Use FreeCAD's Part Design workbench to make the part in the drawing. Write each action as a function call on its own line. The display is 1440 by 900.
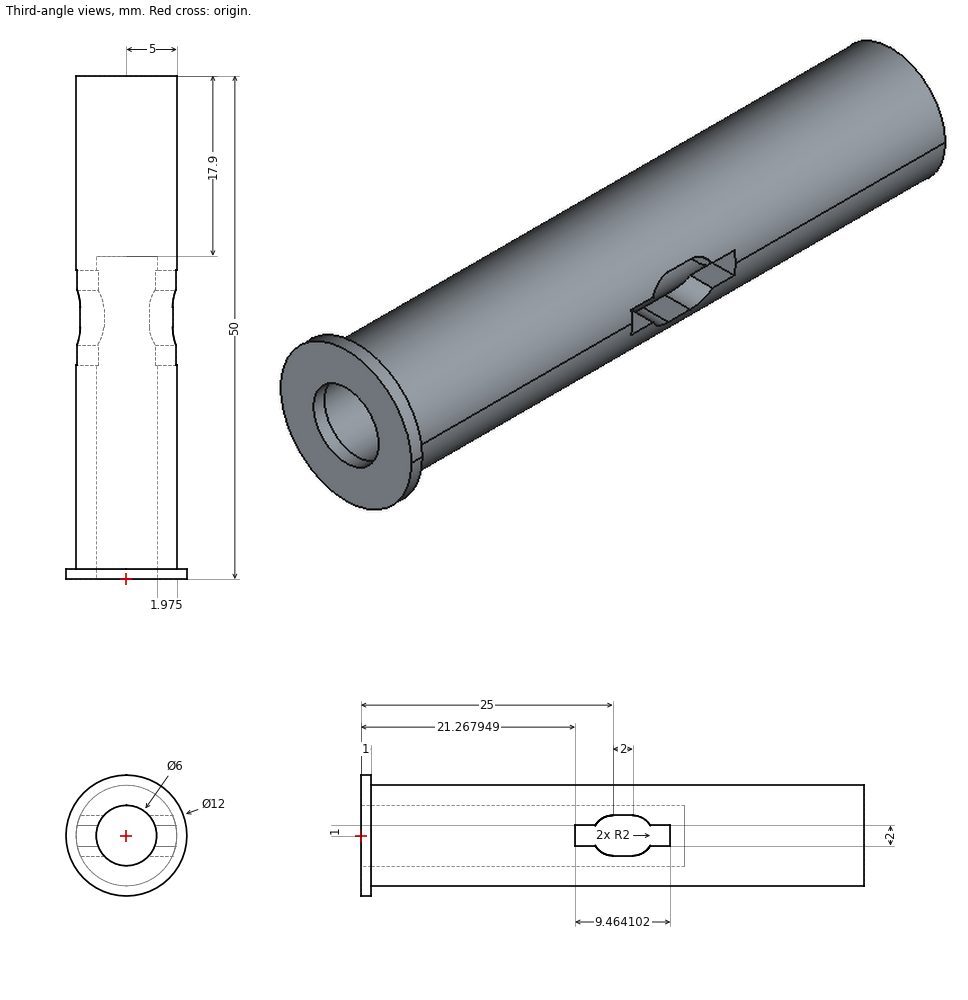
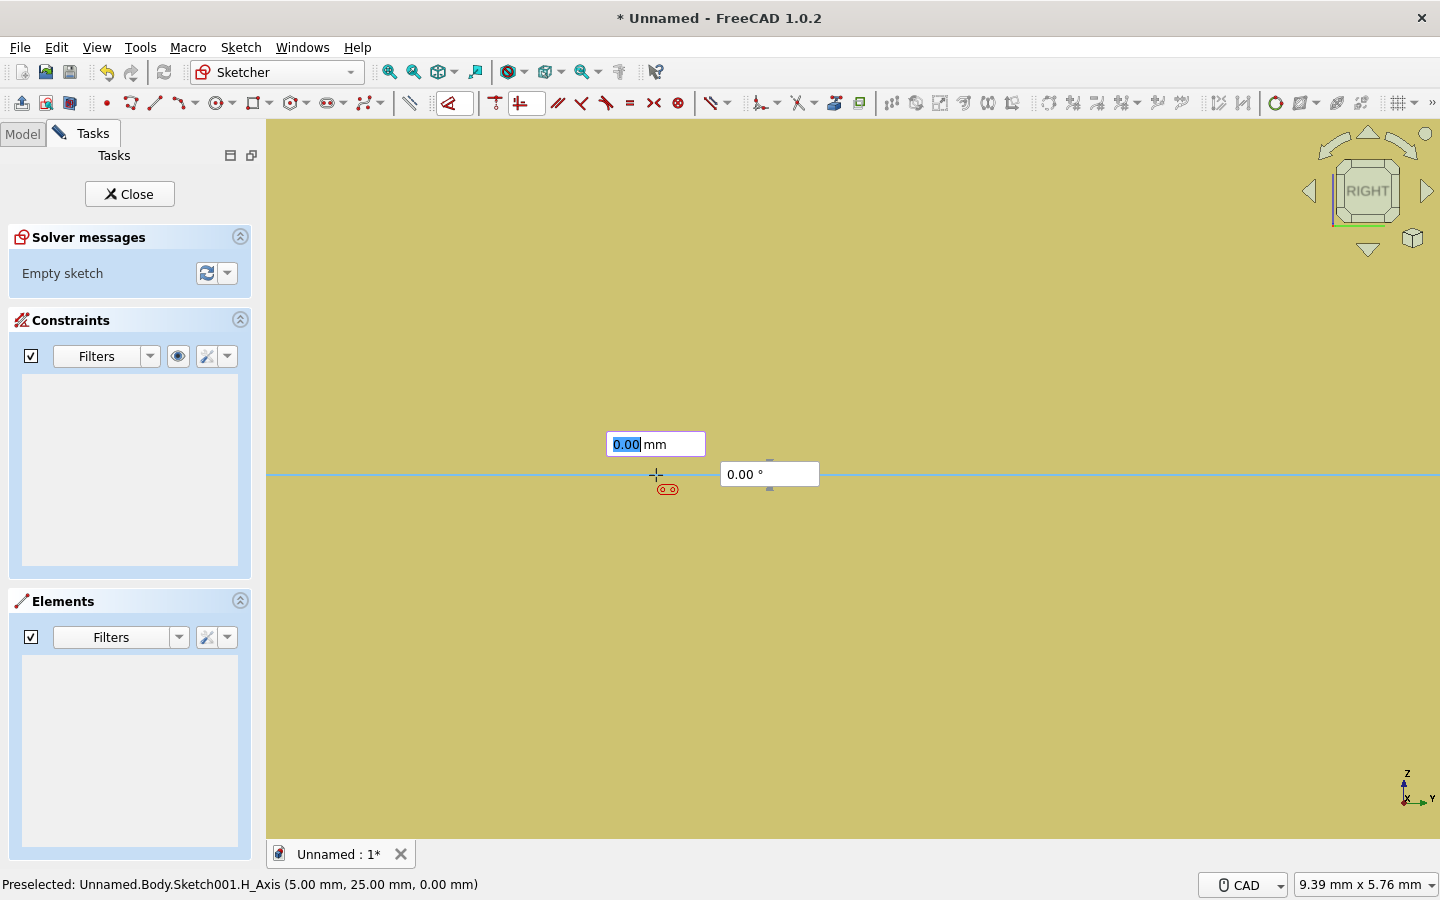
click(906, 466)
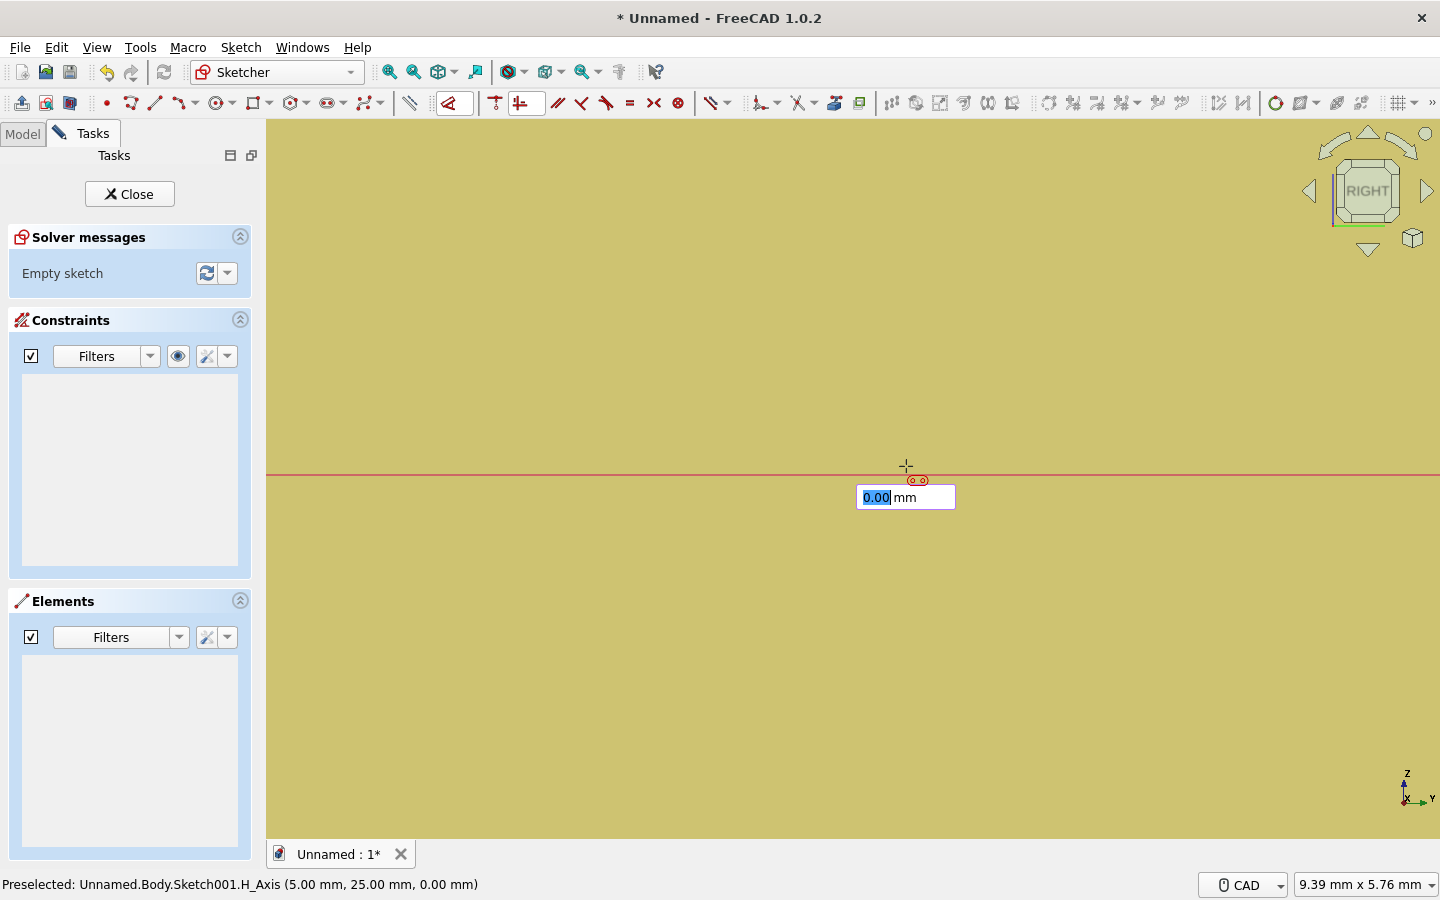
click(781, 725)
key(Escape)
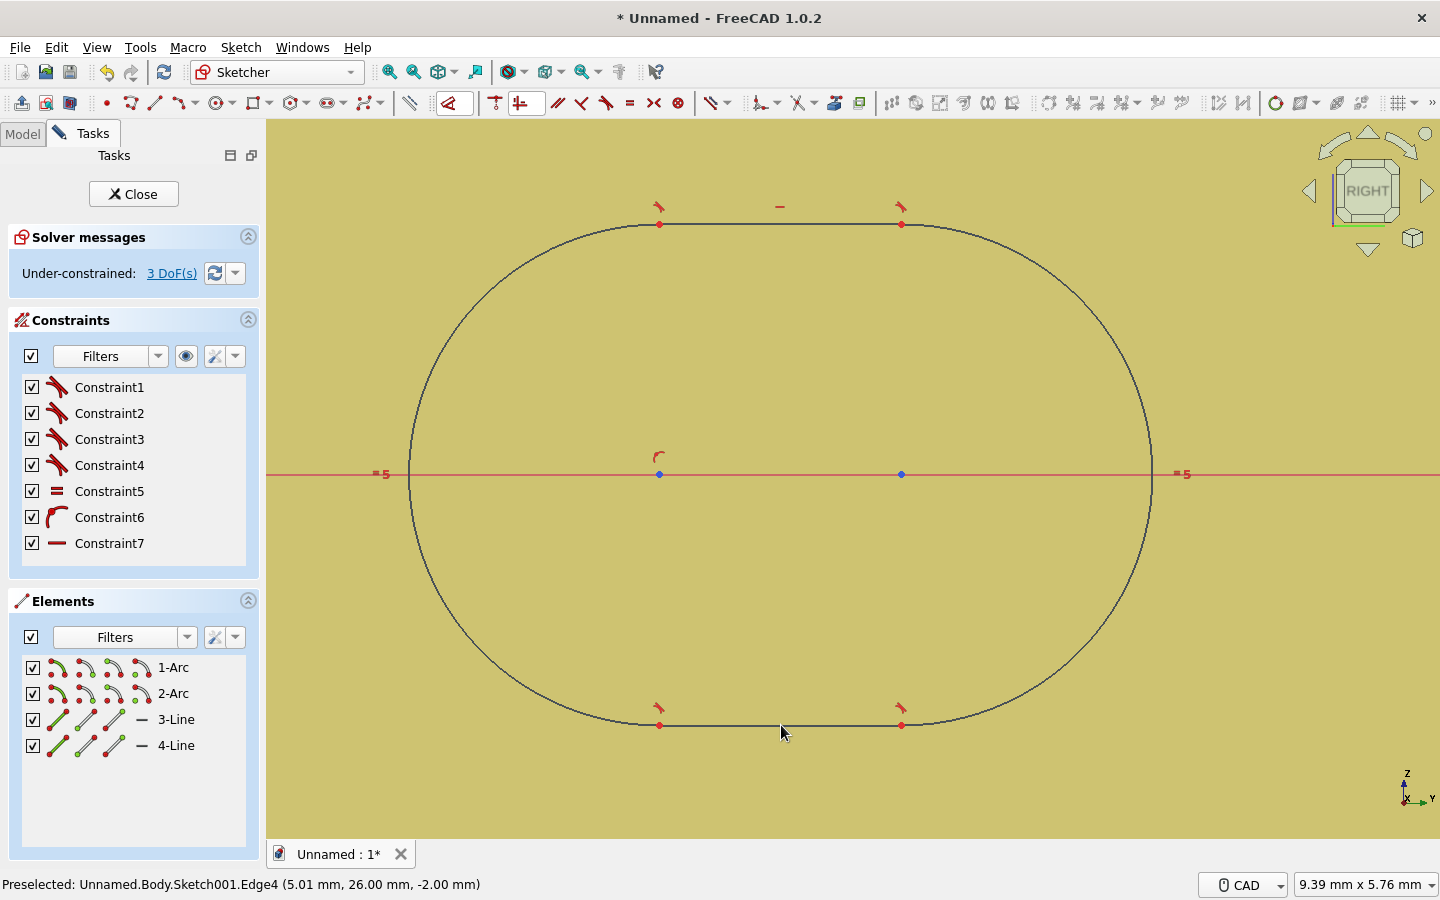
click(457, 328)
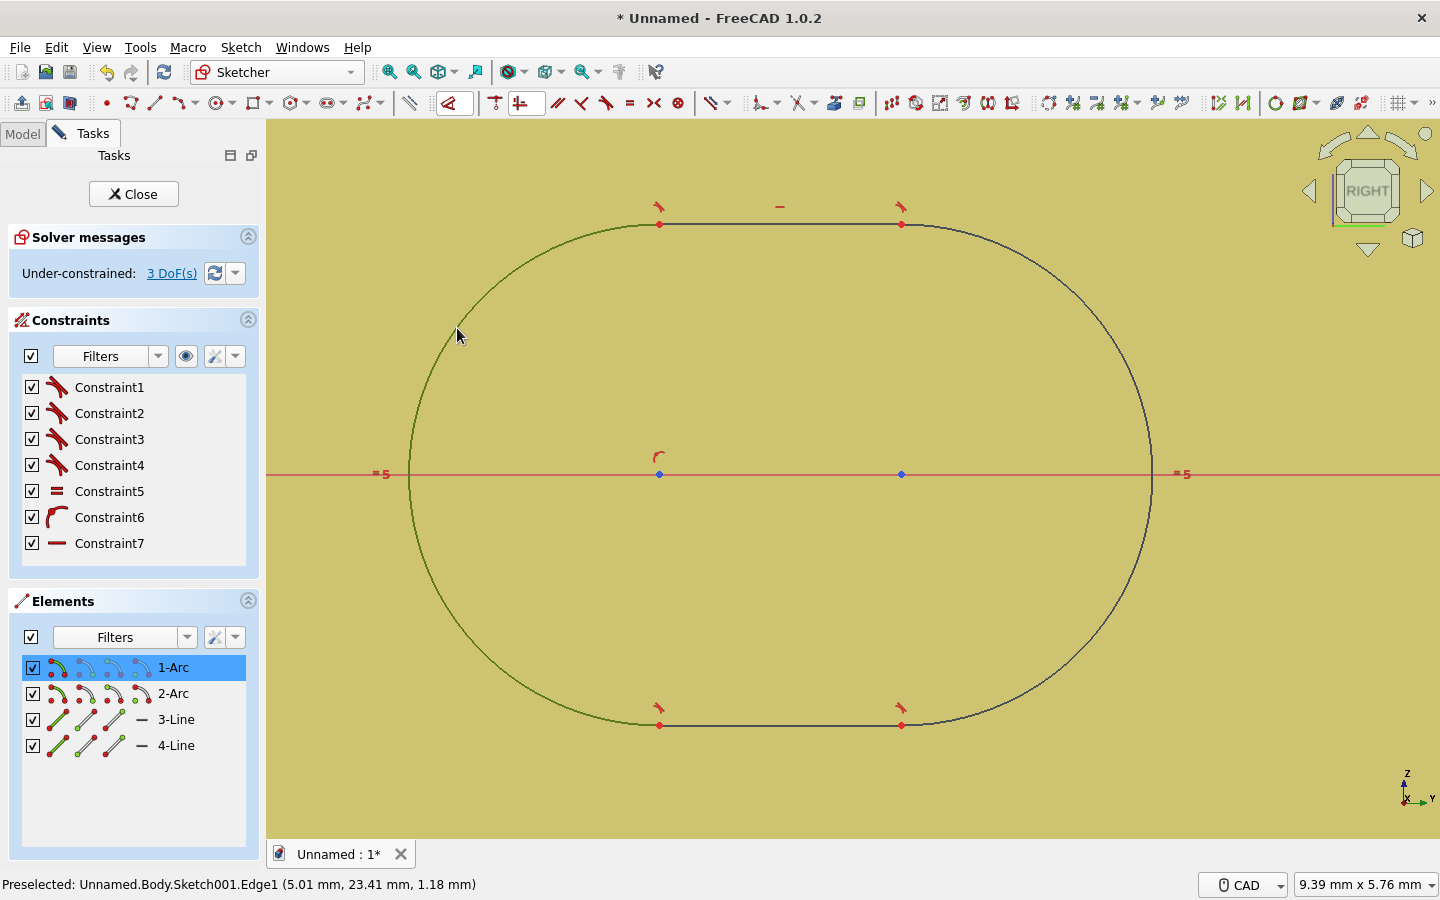
key(k)
key(r)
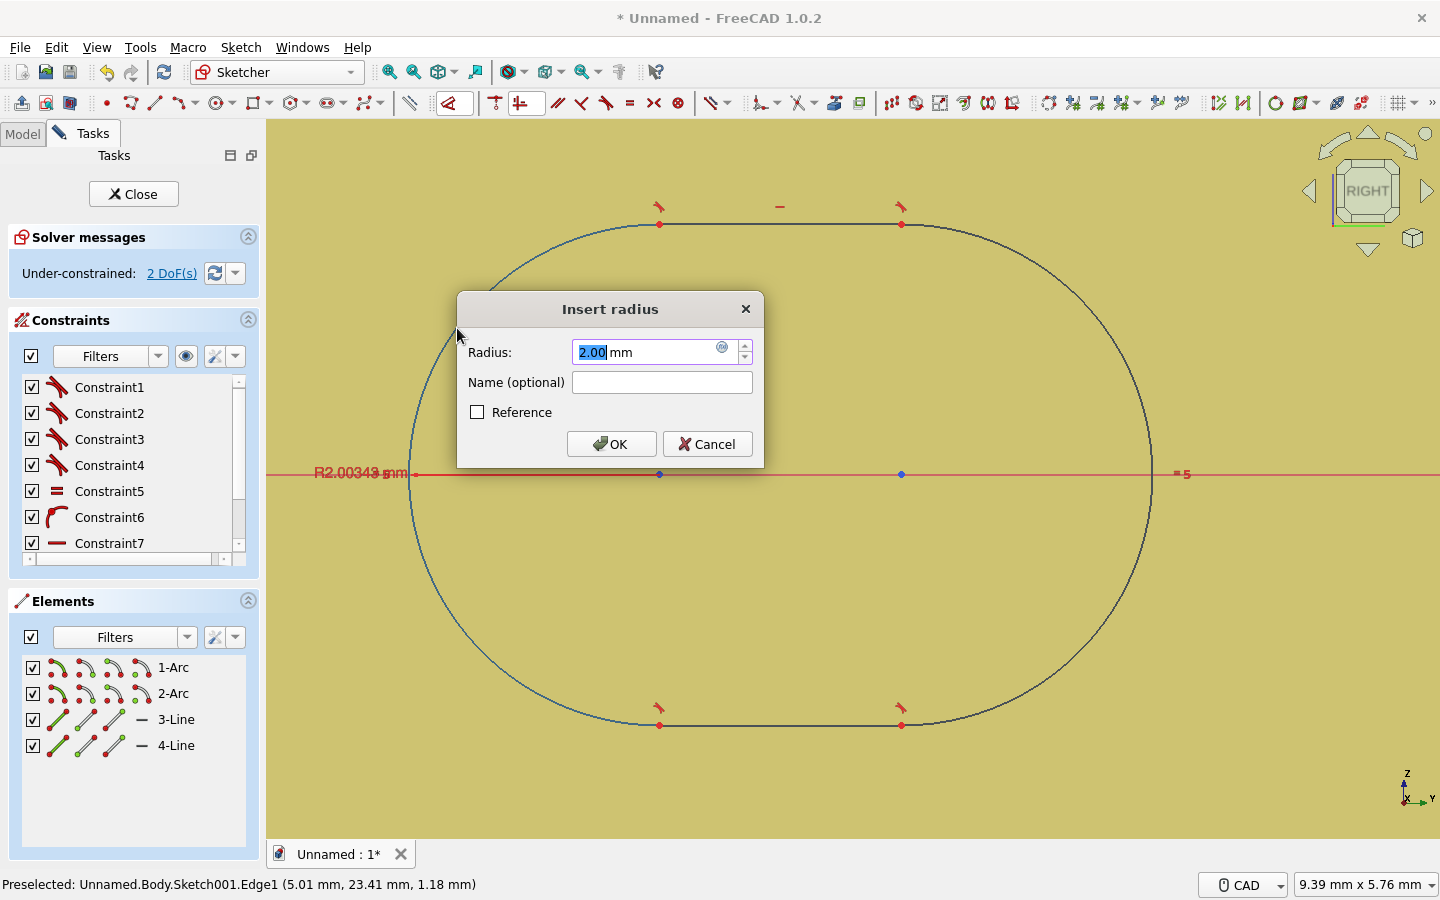
text(2)
key(Return)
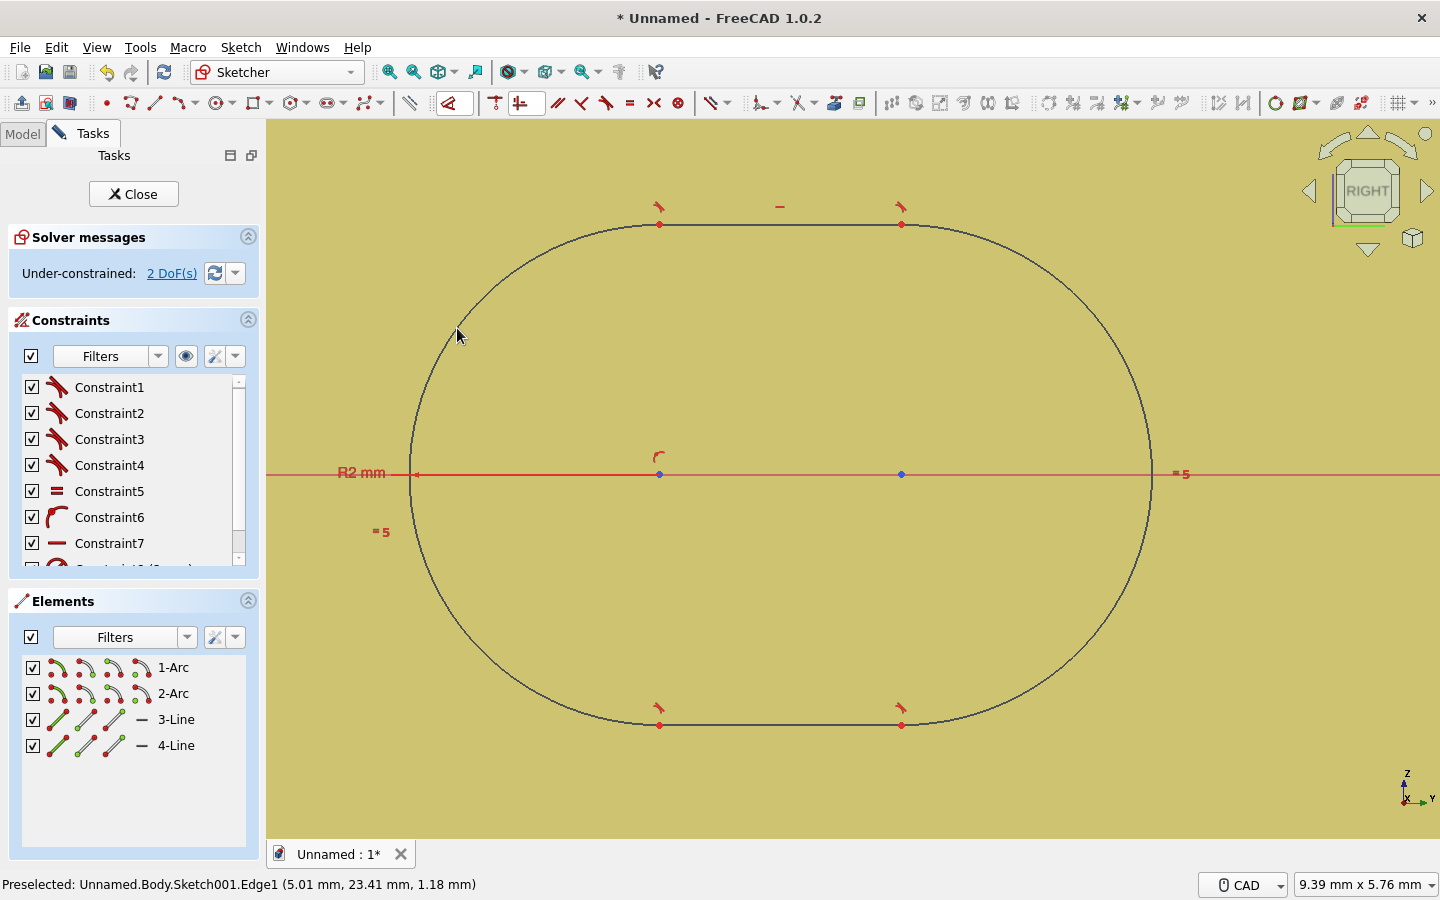
click(732, 225)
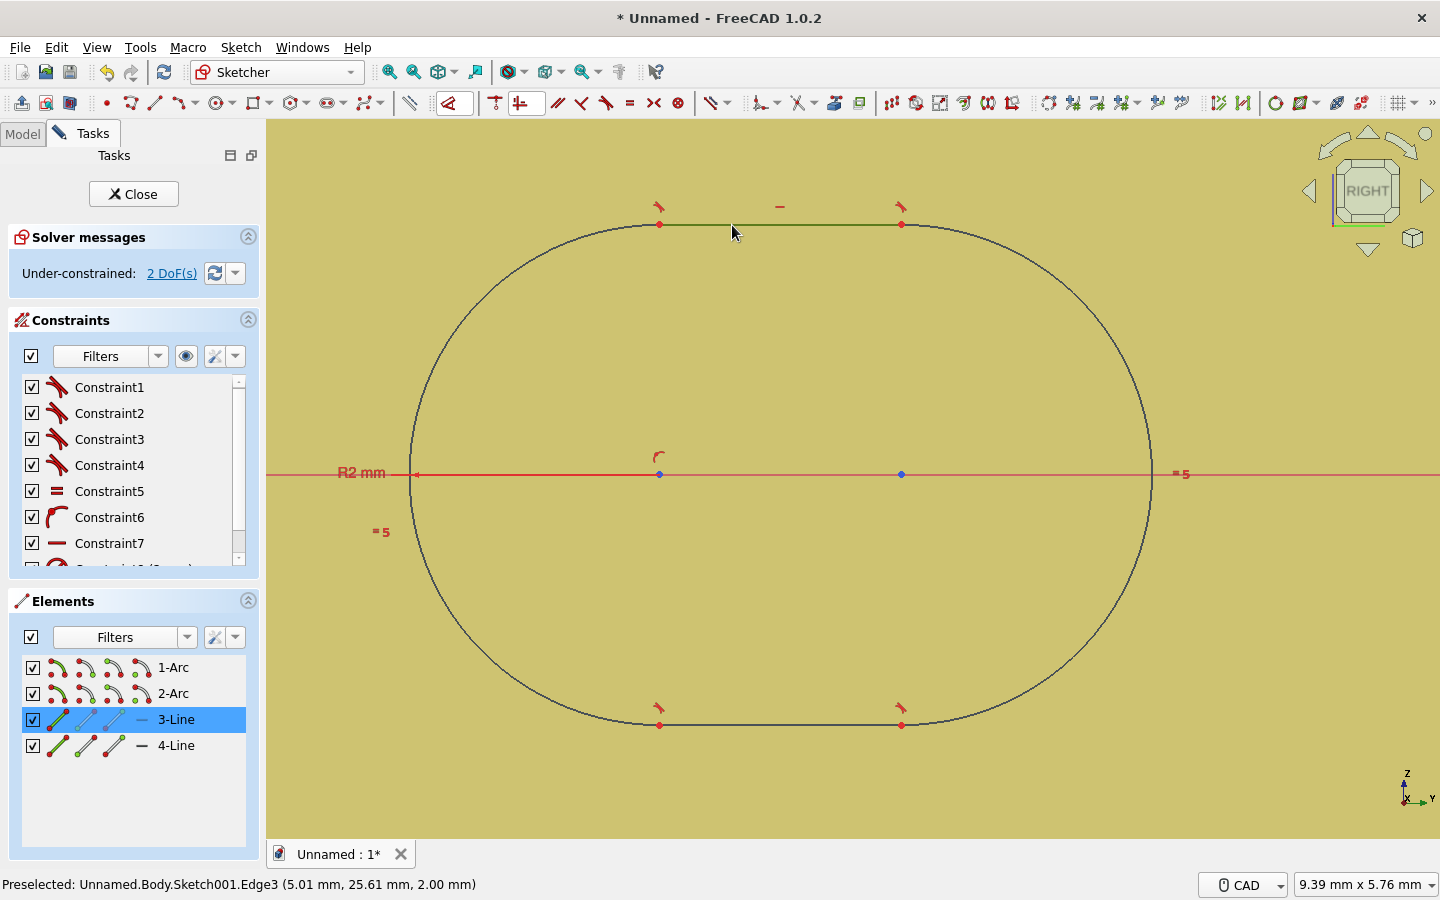
key(l)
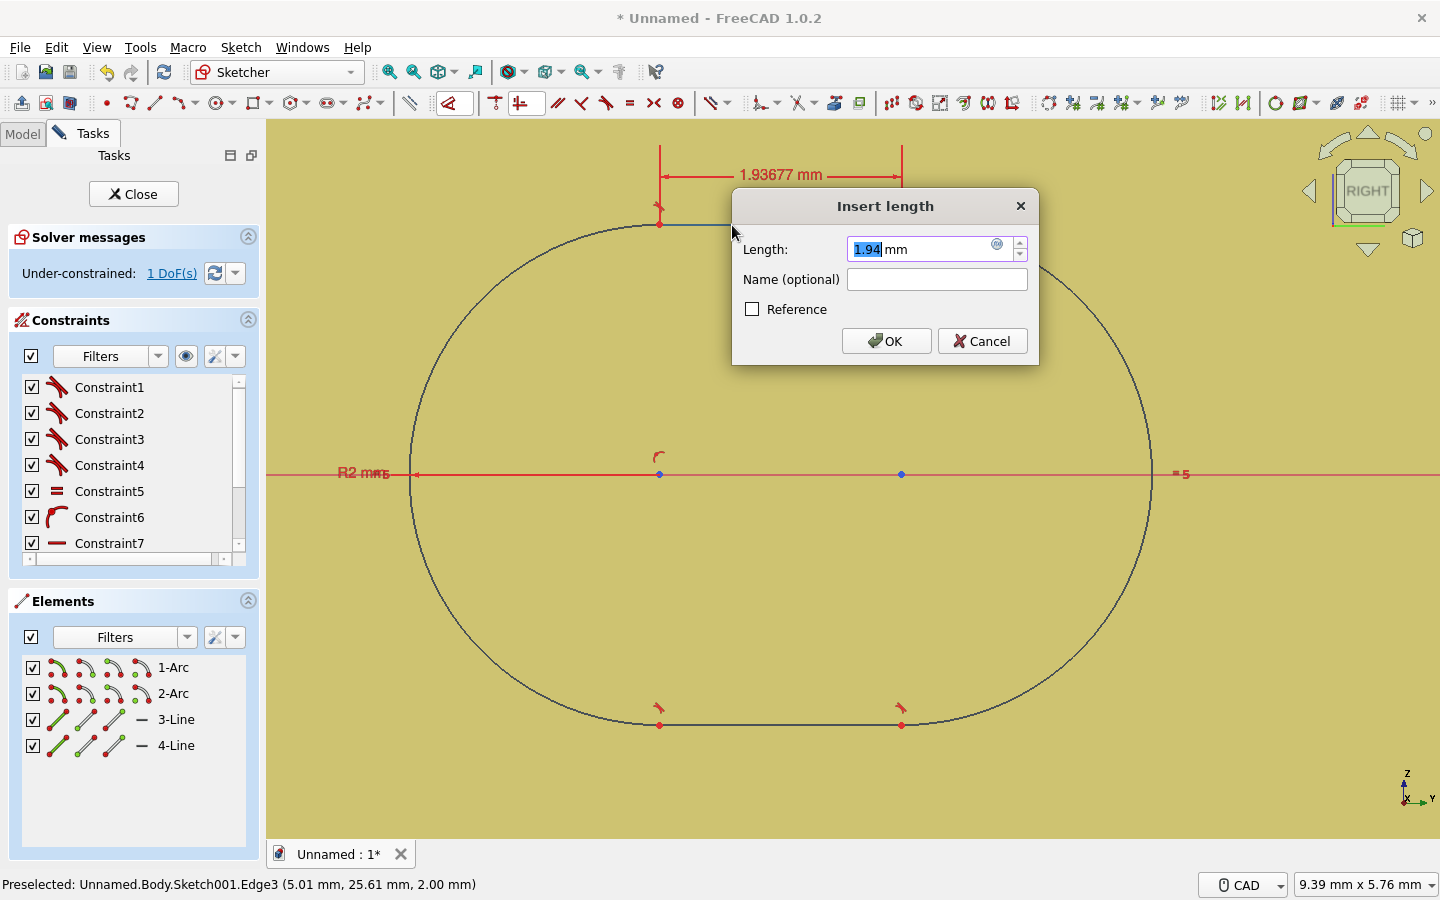
text(2)
key(Return)